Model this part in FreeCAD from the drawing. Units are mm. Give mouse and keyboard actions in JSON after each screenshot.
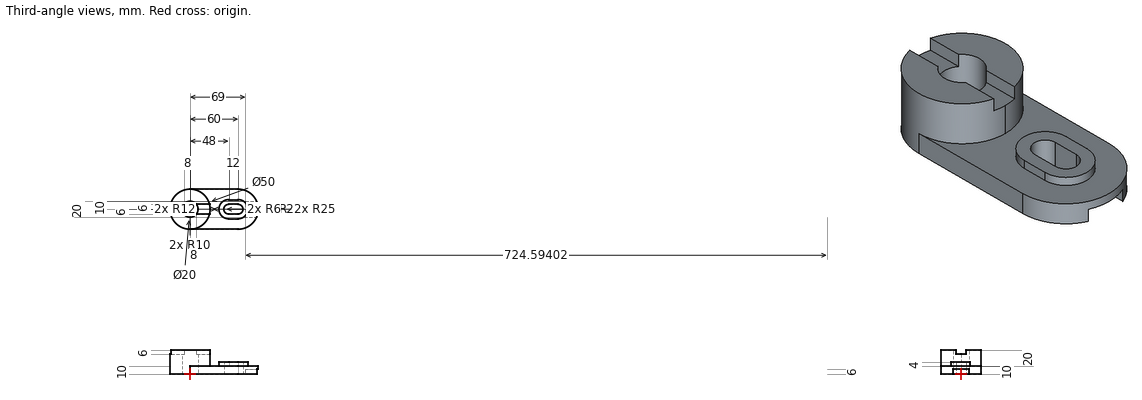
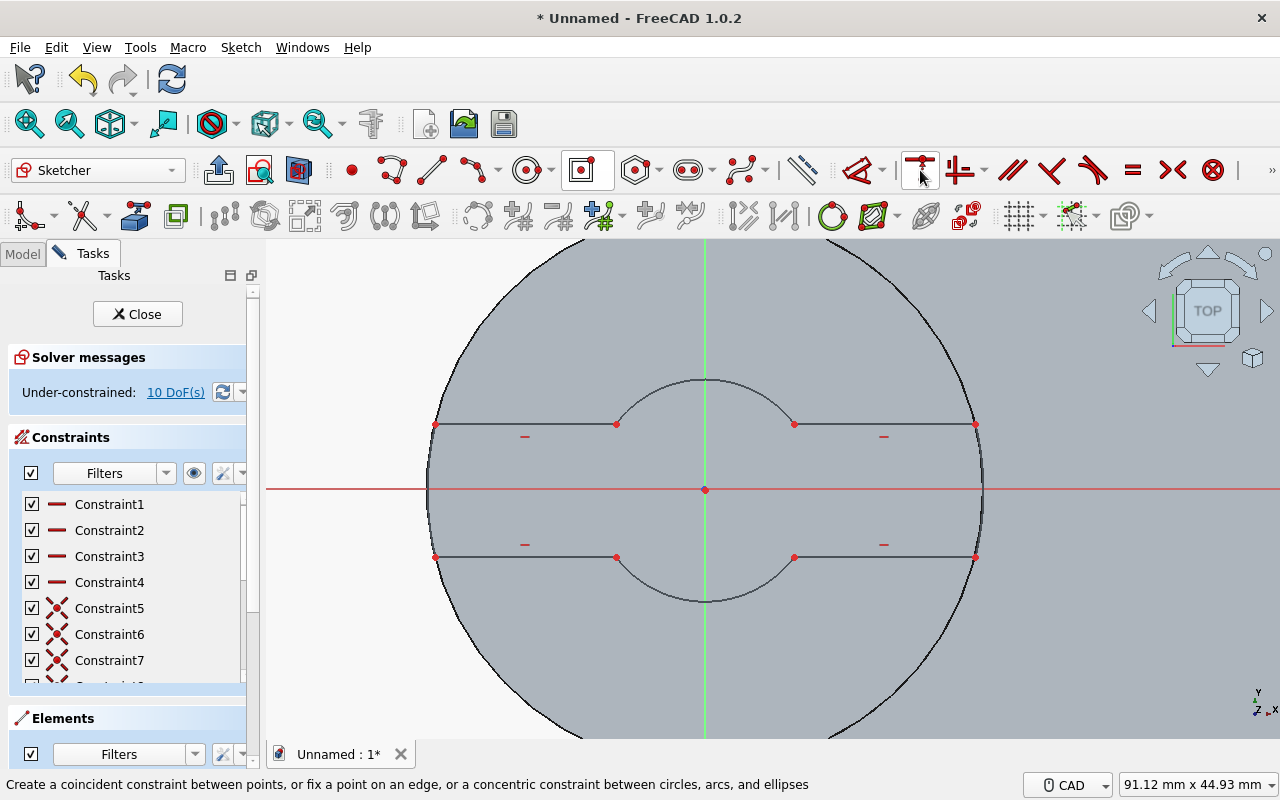
{"action": "left_click_drag", "start_coordinate": [695, 479], "coordinate": [715, 501]}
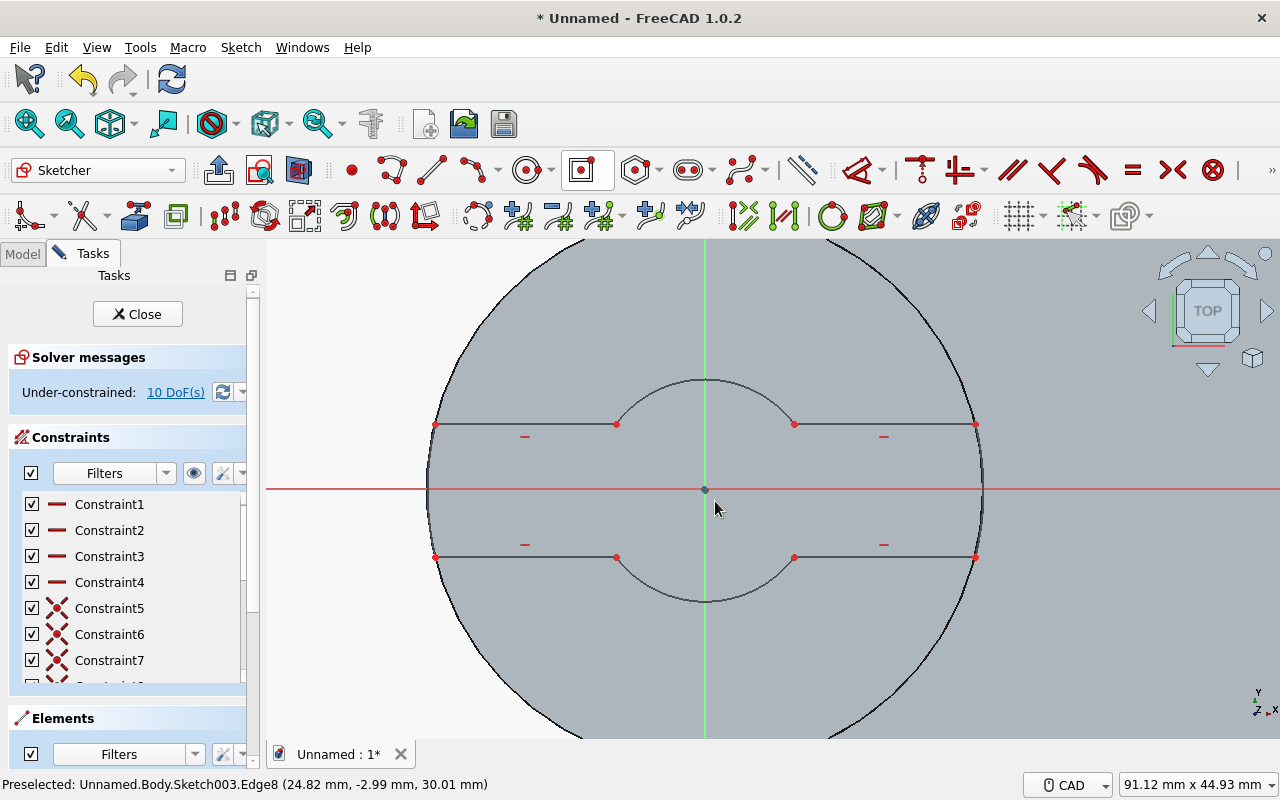
{"action": "left_click", "coordinate": [920, 170]}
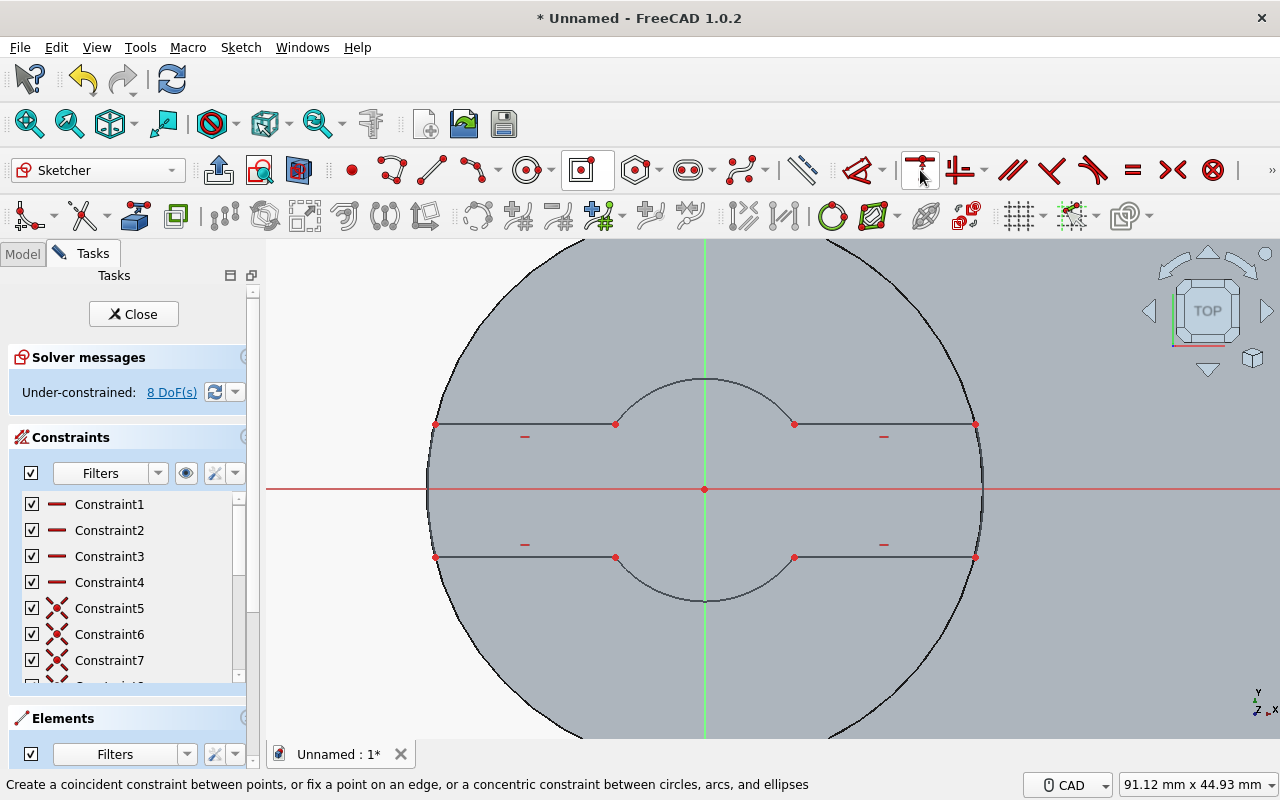
{"action": "left_click", "coordinate": [745, 386]}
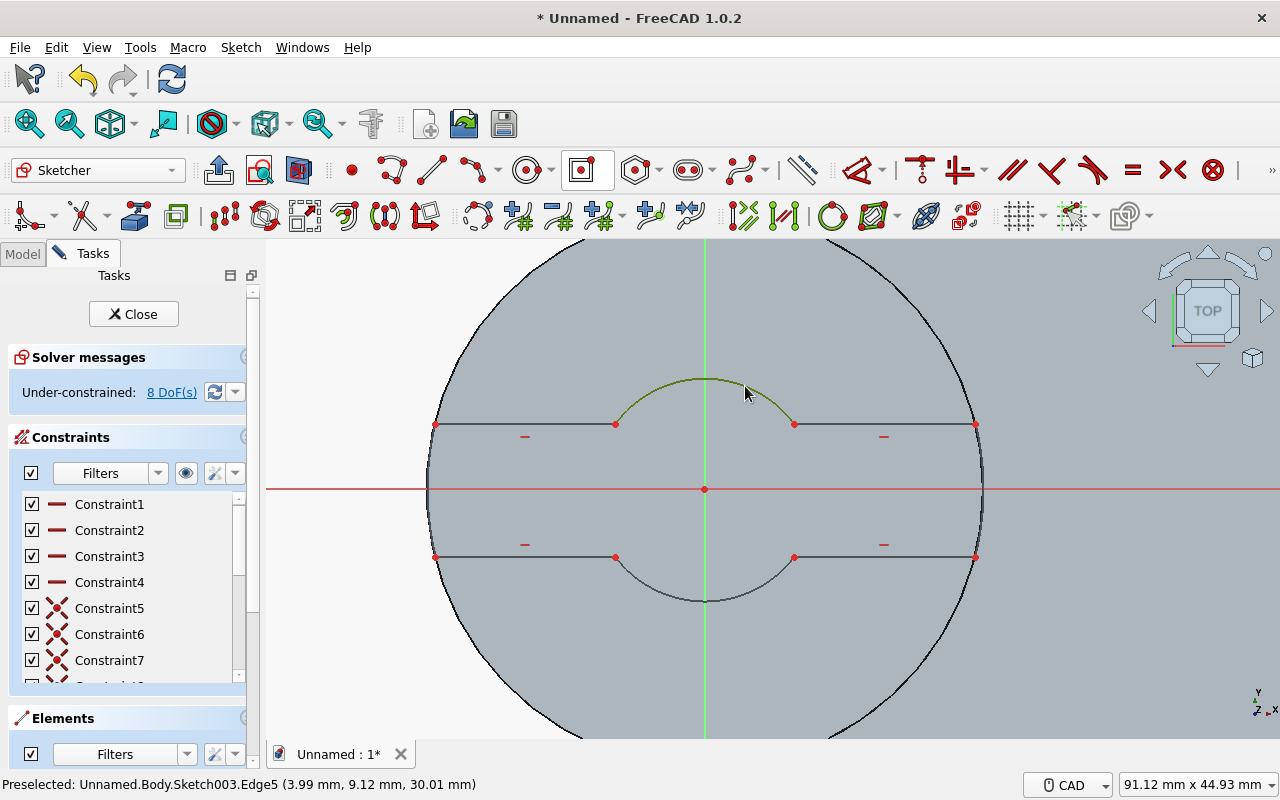
{"action": "left_click", "coordinate": [664, 594]}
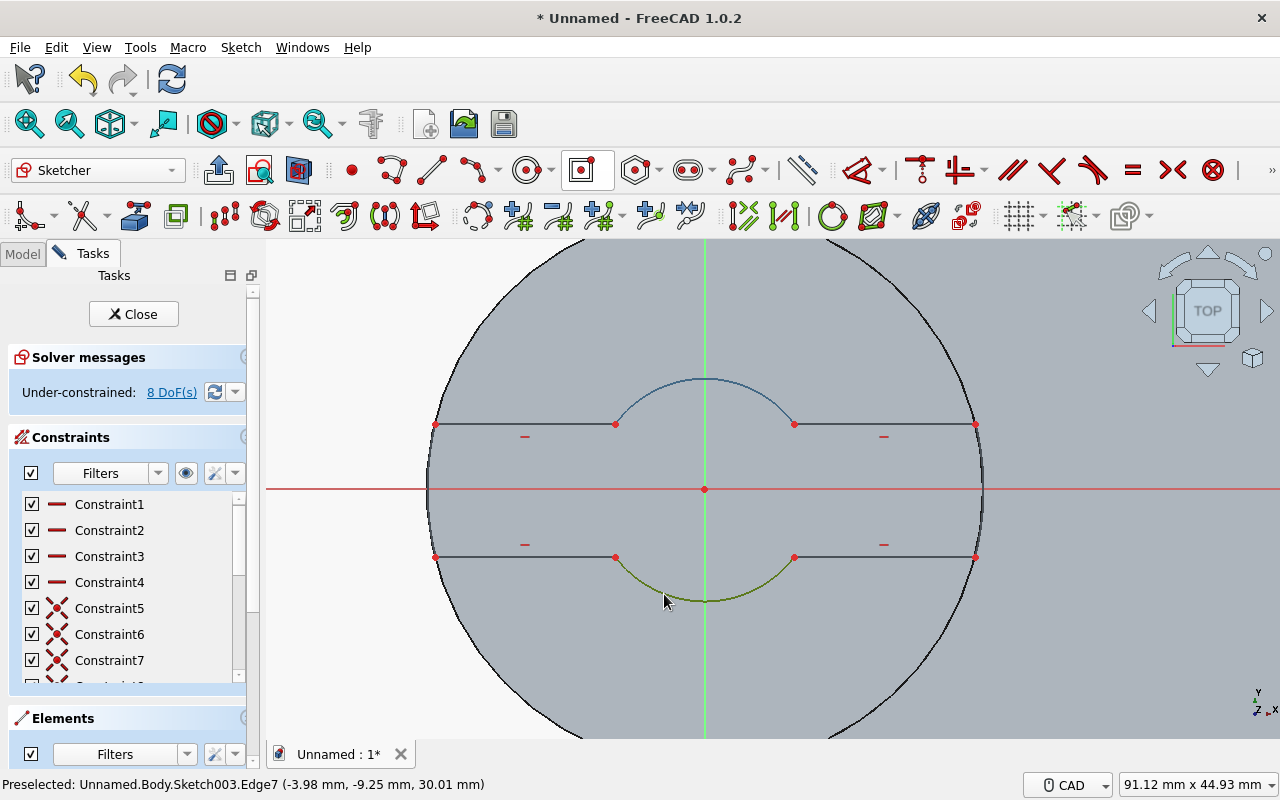
{"action": "left_click", "coordinate": [1134, 170]}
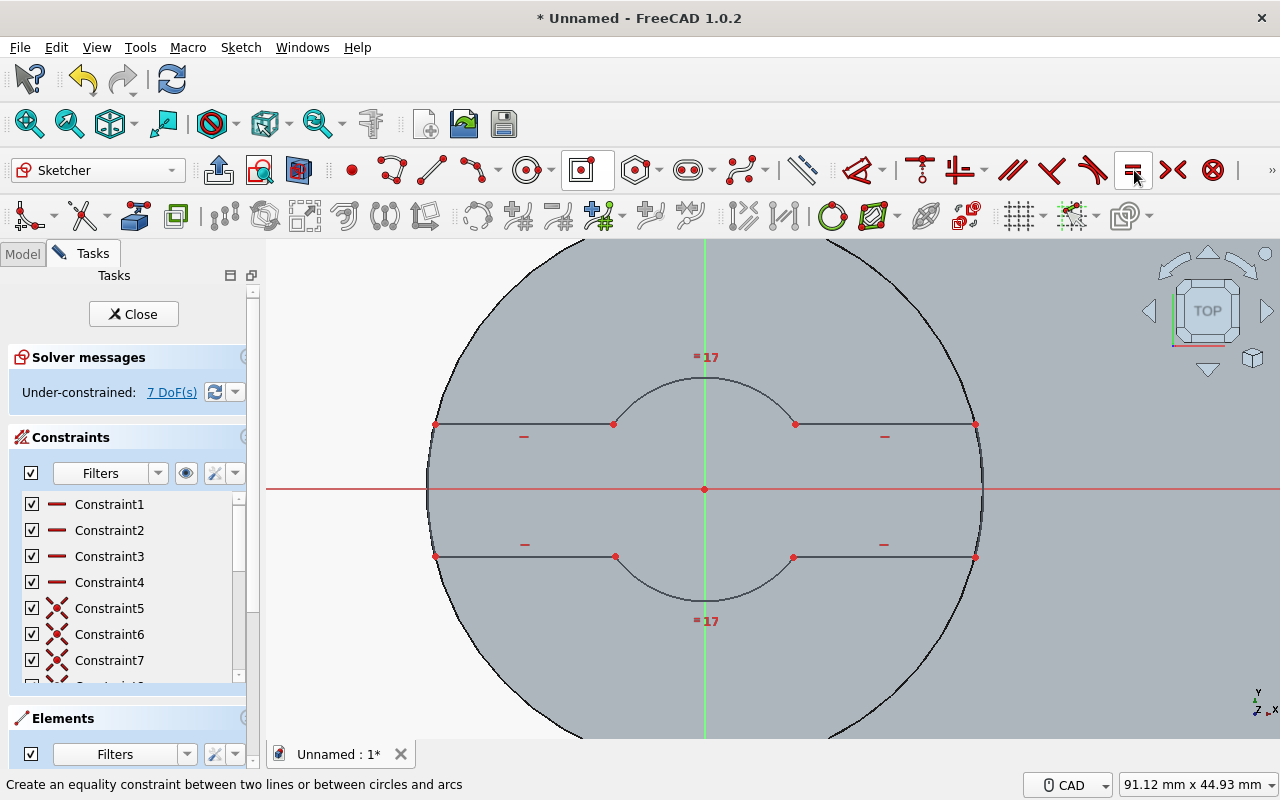
{"action": "left_click", "coordinate": [429, 464]}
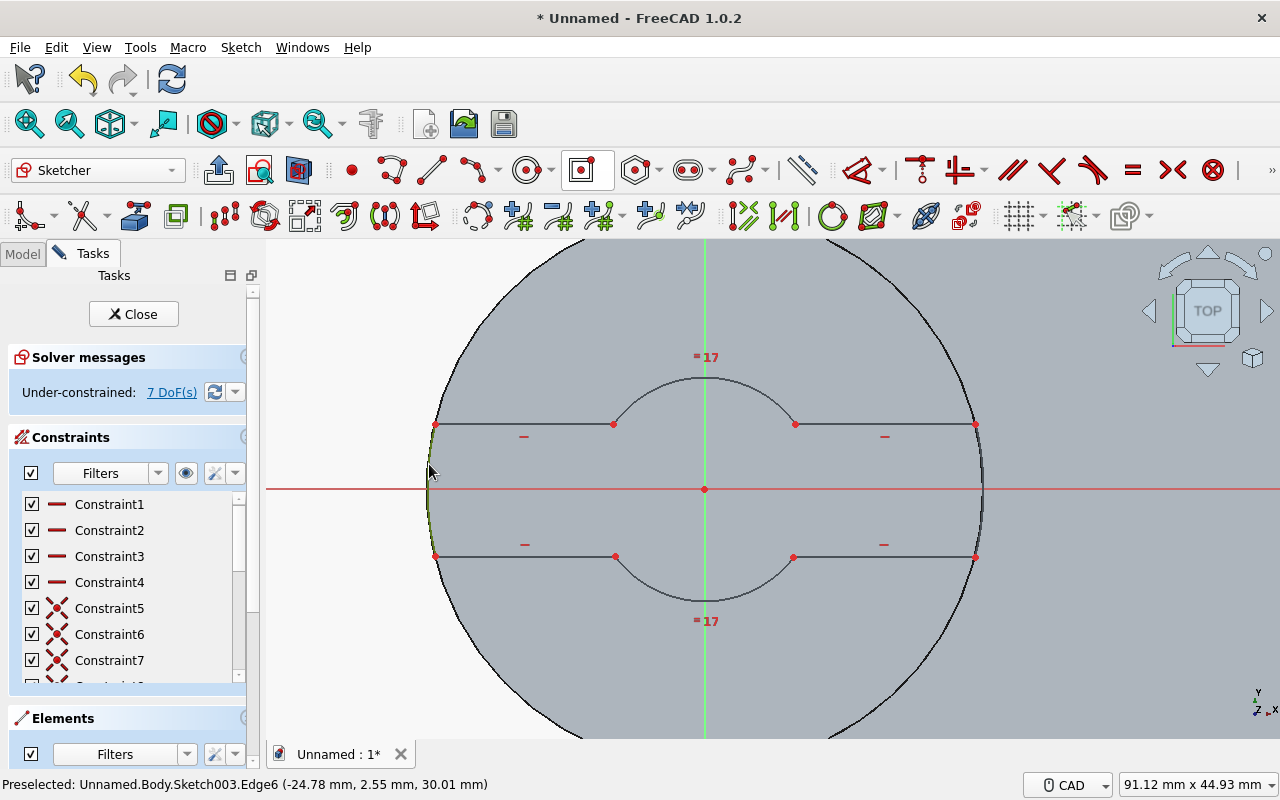
{"action": "left_click", "coordinate": [982, 517]}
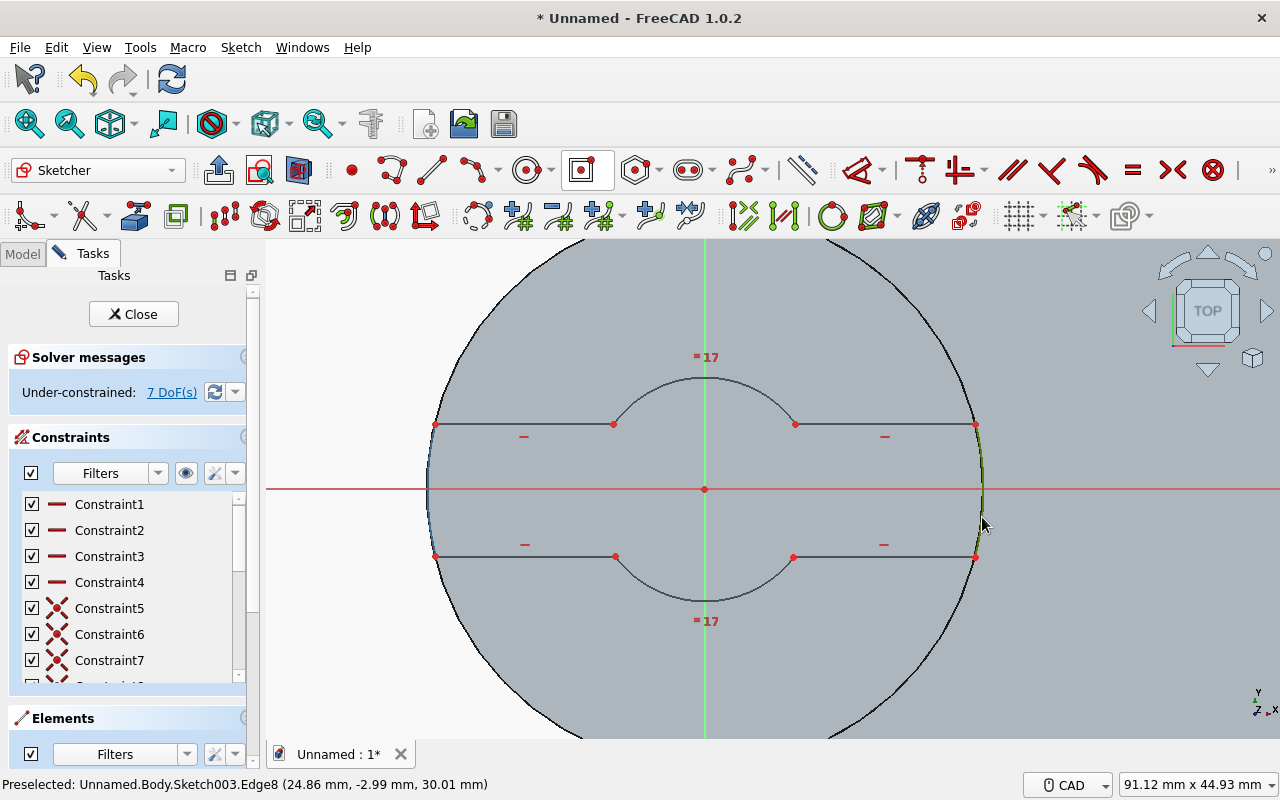
{"action": "left_click", "coordinate": [1134, 170]}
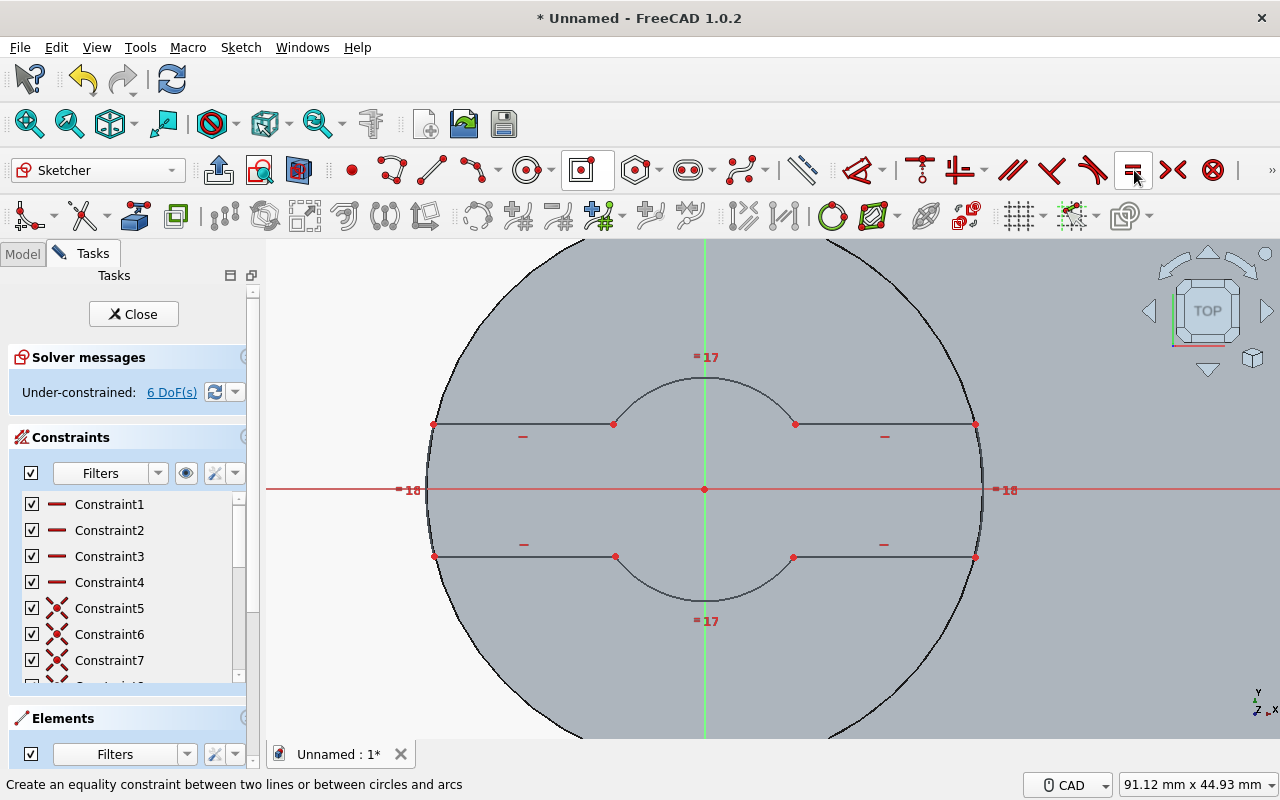
{"action": "left_click", "coordinate": [858, 170]}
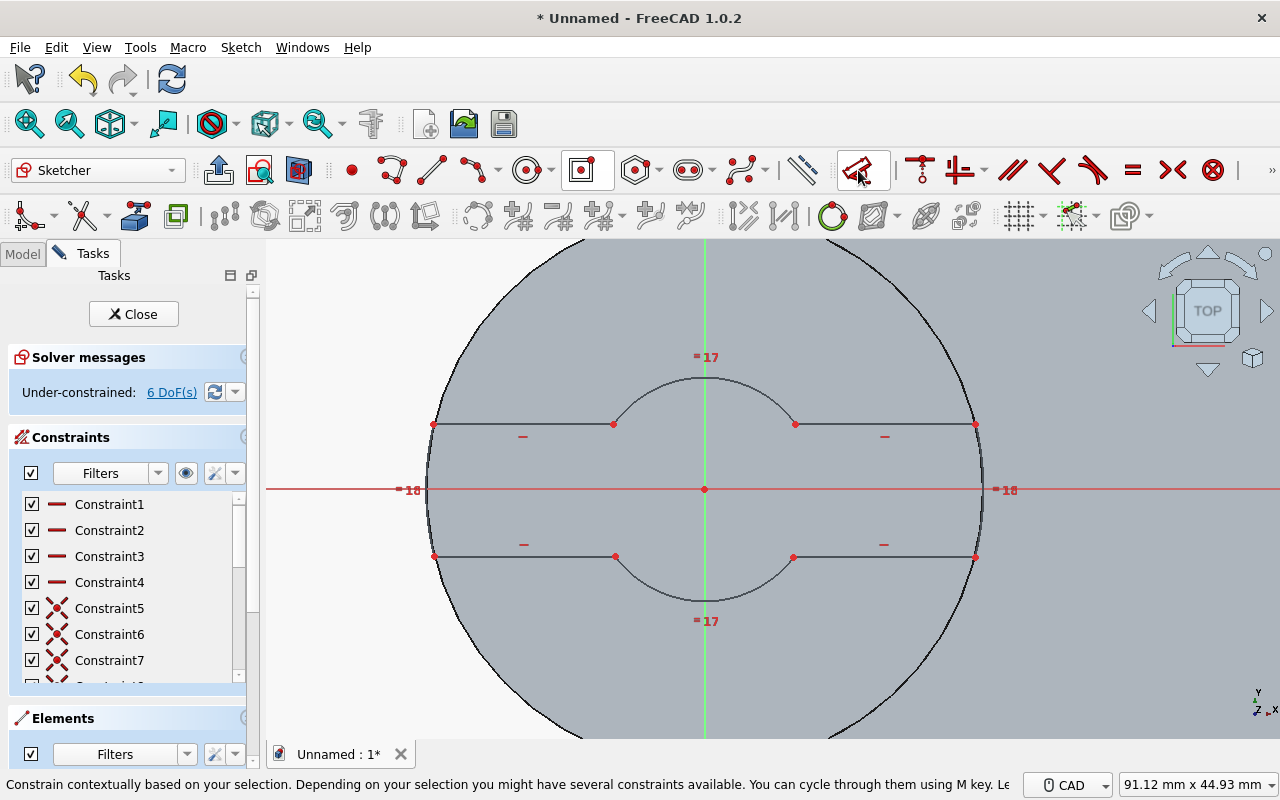
{"action": "left_click", "coordinate": [746, 385]}
{"action": "left_click", "coordinate": [758, 355]}